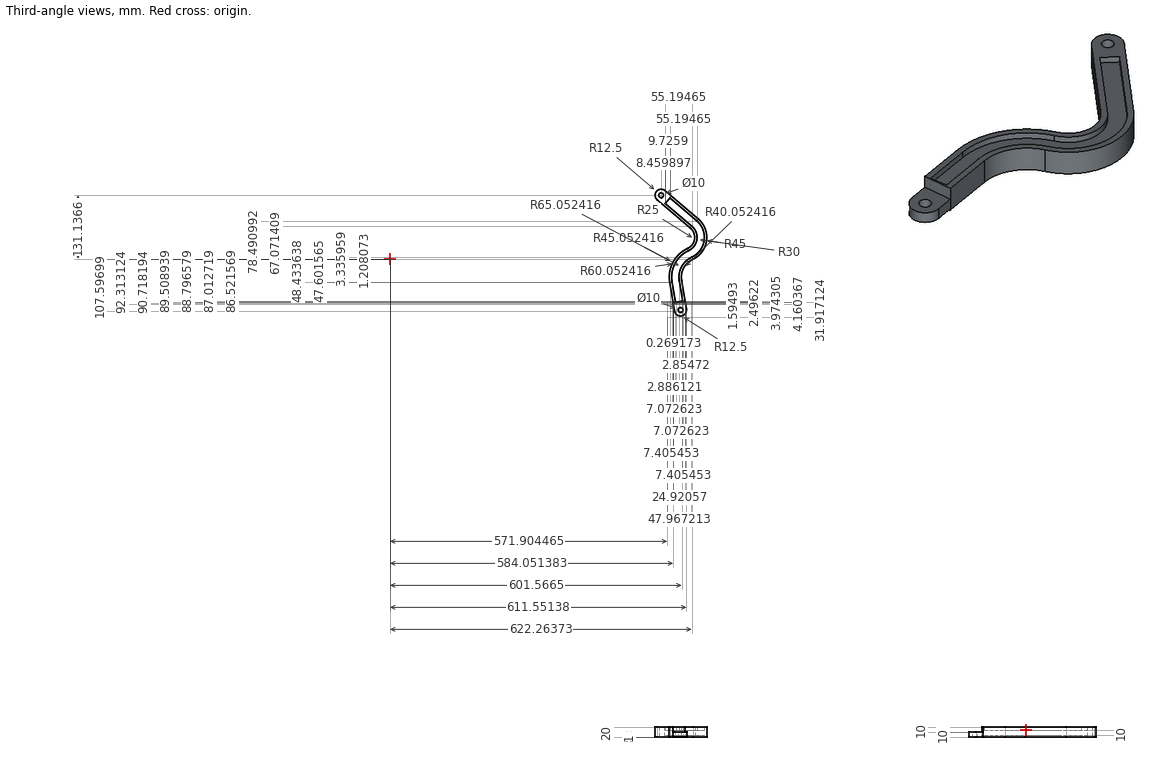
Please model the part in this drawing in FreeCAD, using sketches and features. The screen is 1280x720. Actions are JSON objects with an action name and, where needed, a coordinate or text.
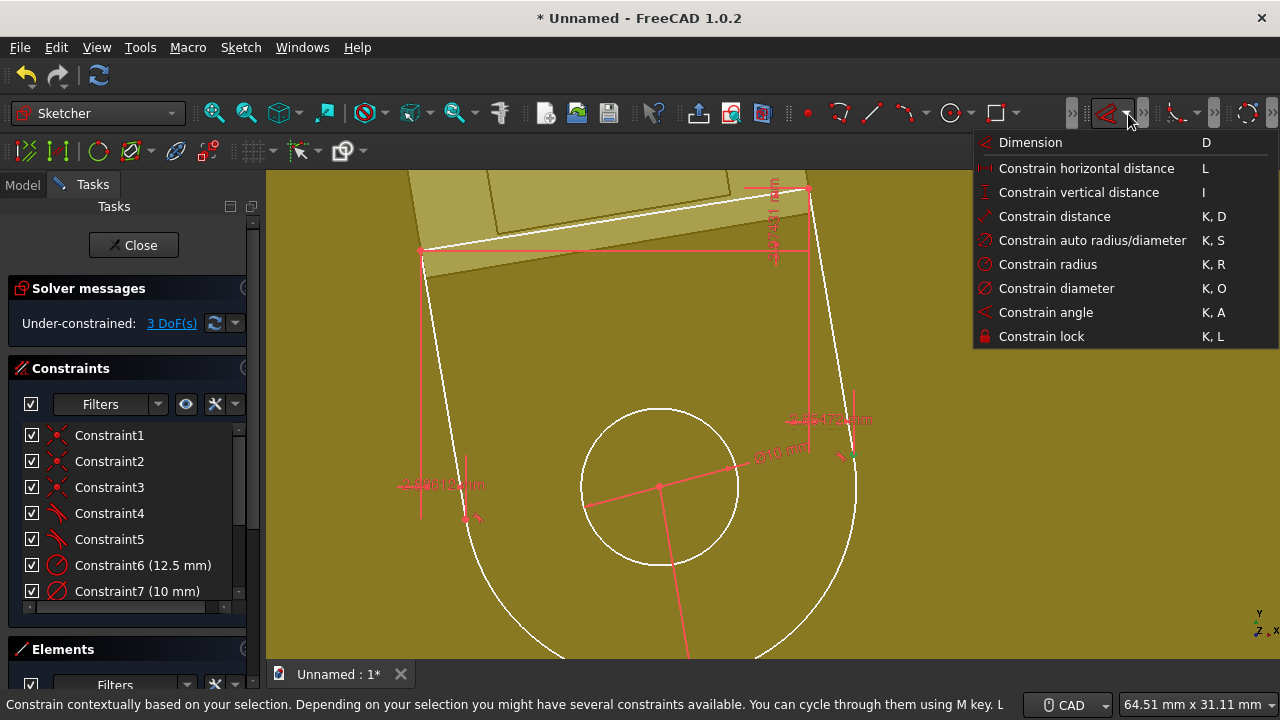
{"action": "left_click", "coordinate": [1126, 168]}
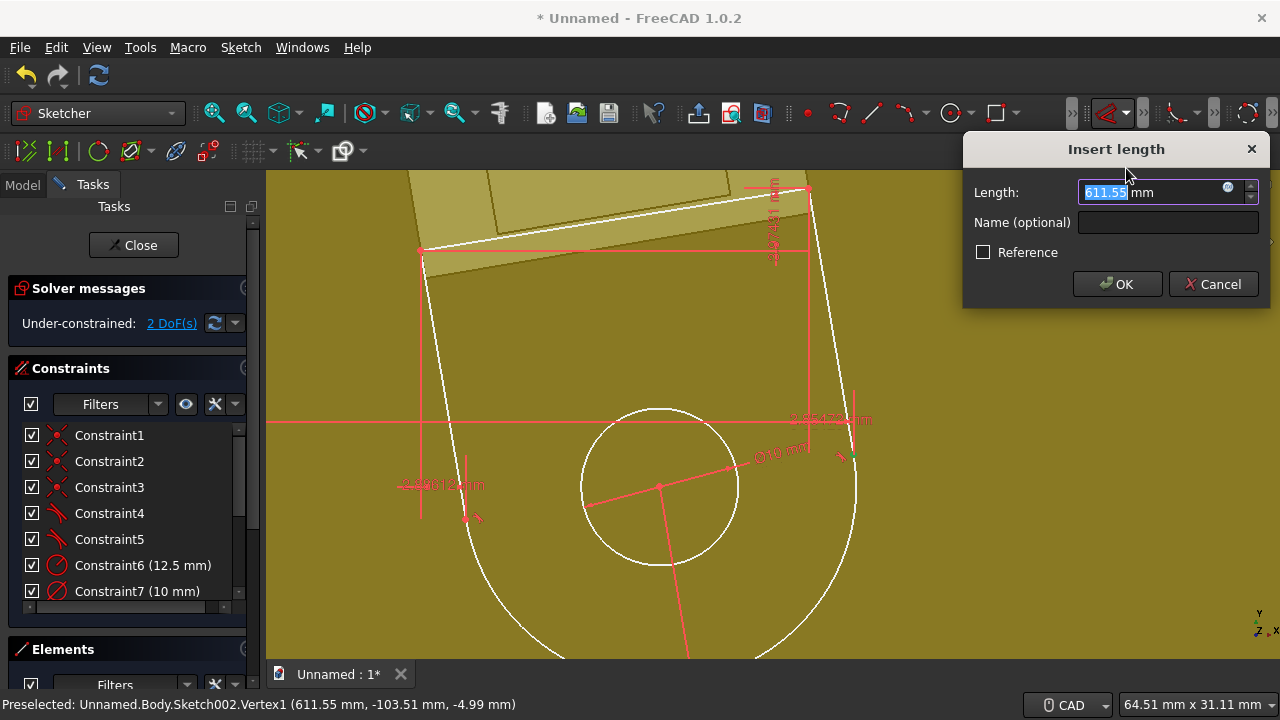
{"action": "type", "text": "611.55138"}
{"action": "key", "text": "Return"}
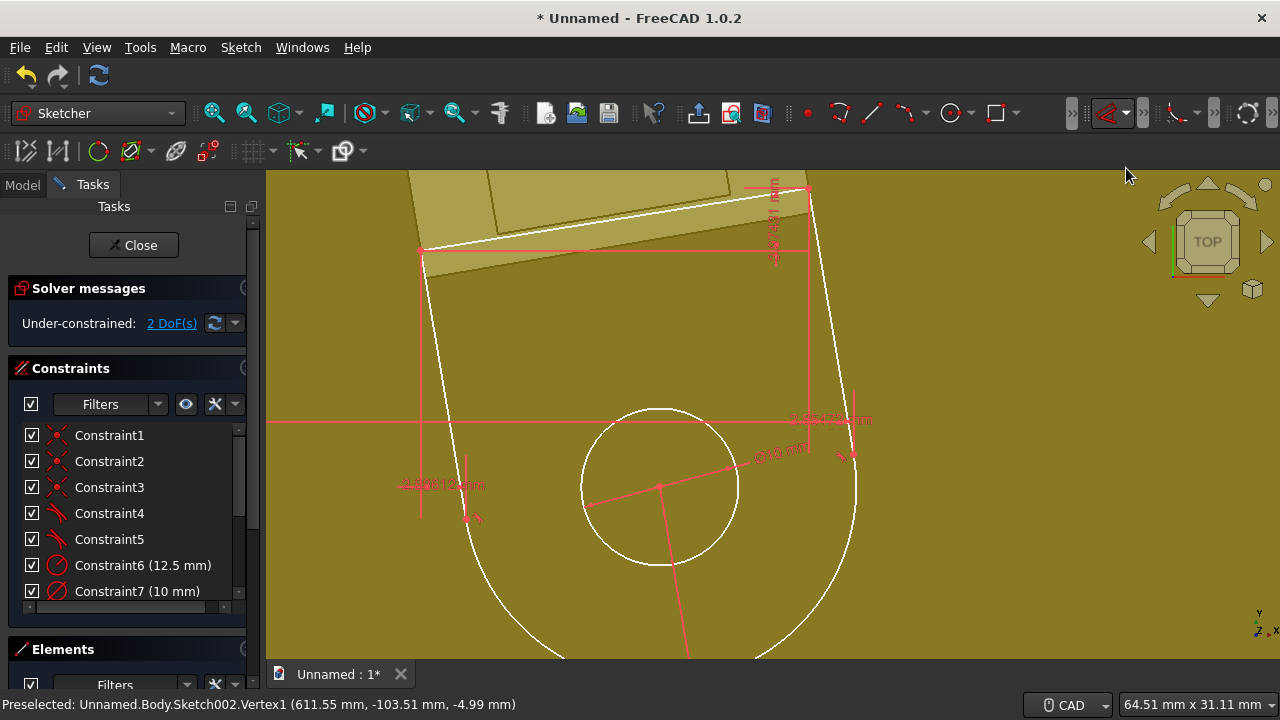
{"action": "scroll", "coordinate": [841, 376], "scroll_direction": "down", "scroll_amount": 2}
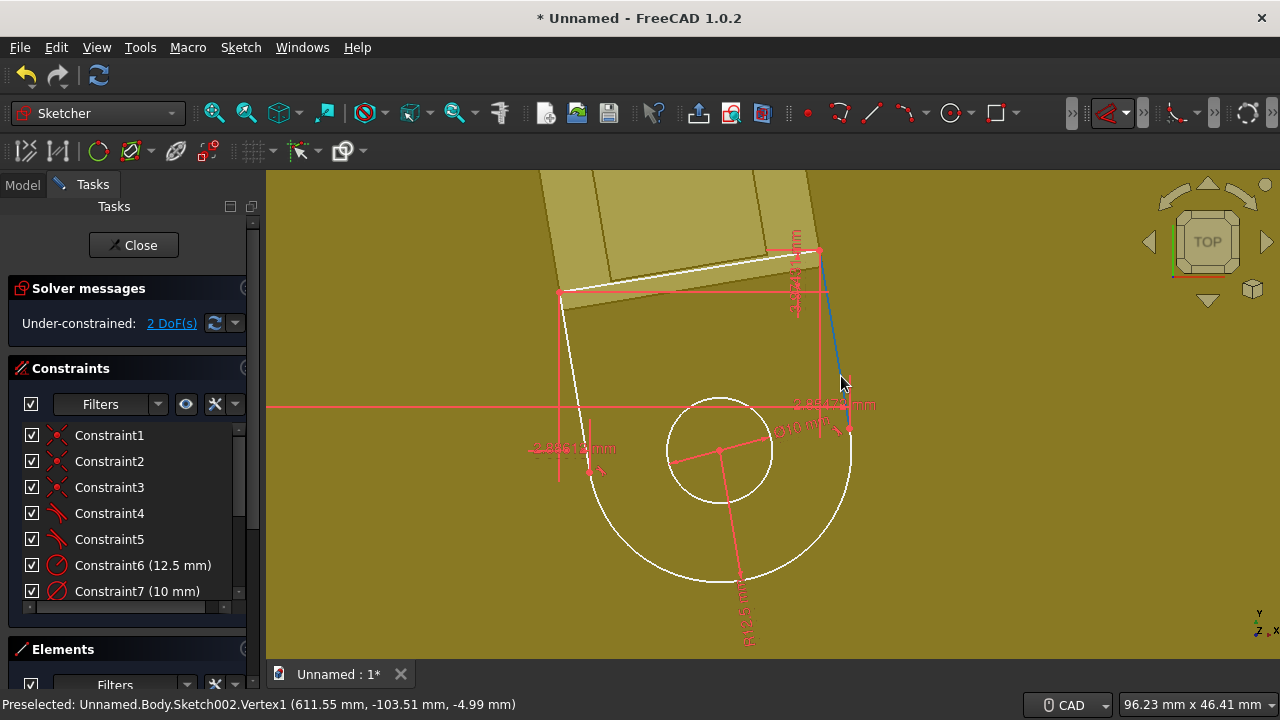
{"action": "left_click", "coordinate": [820, 250]}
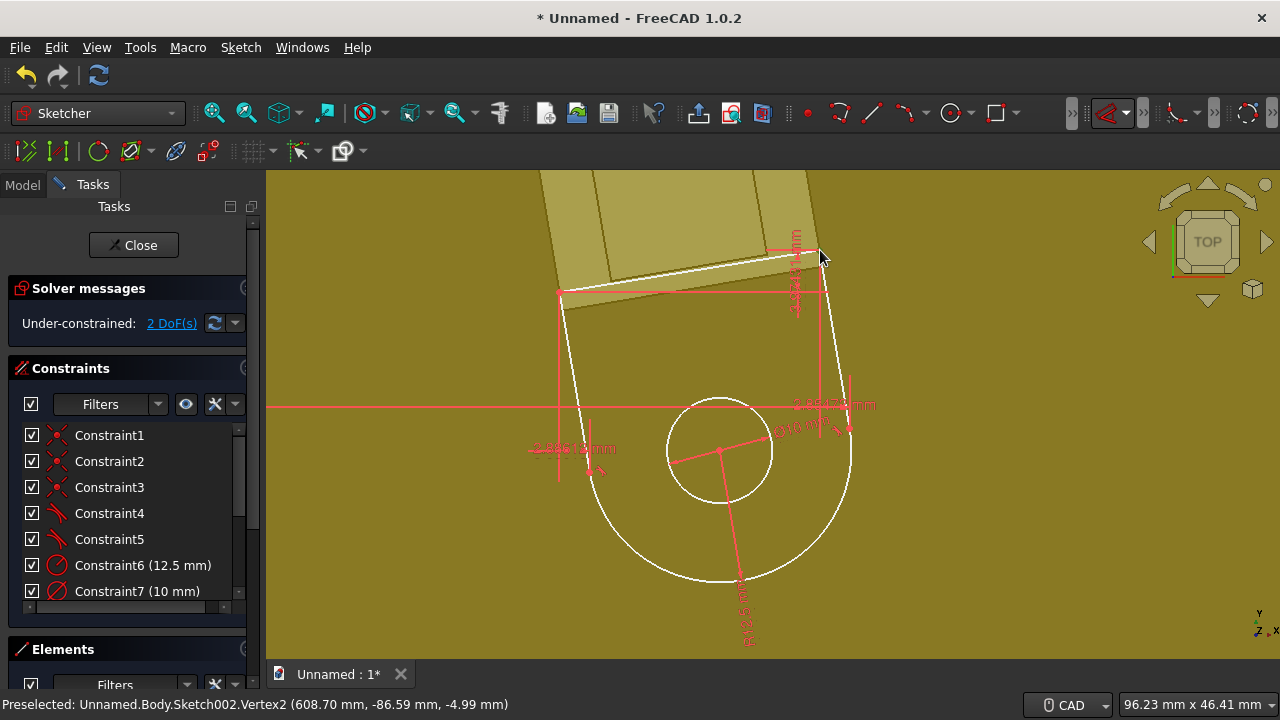
{"action": "key", "text": "i"}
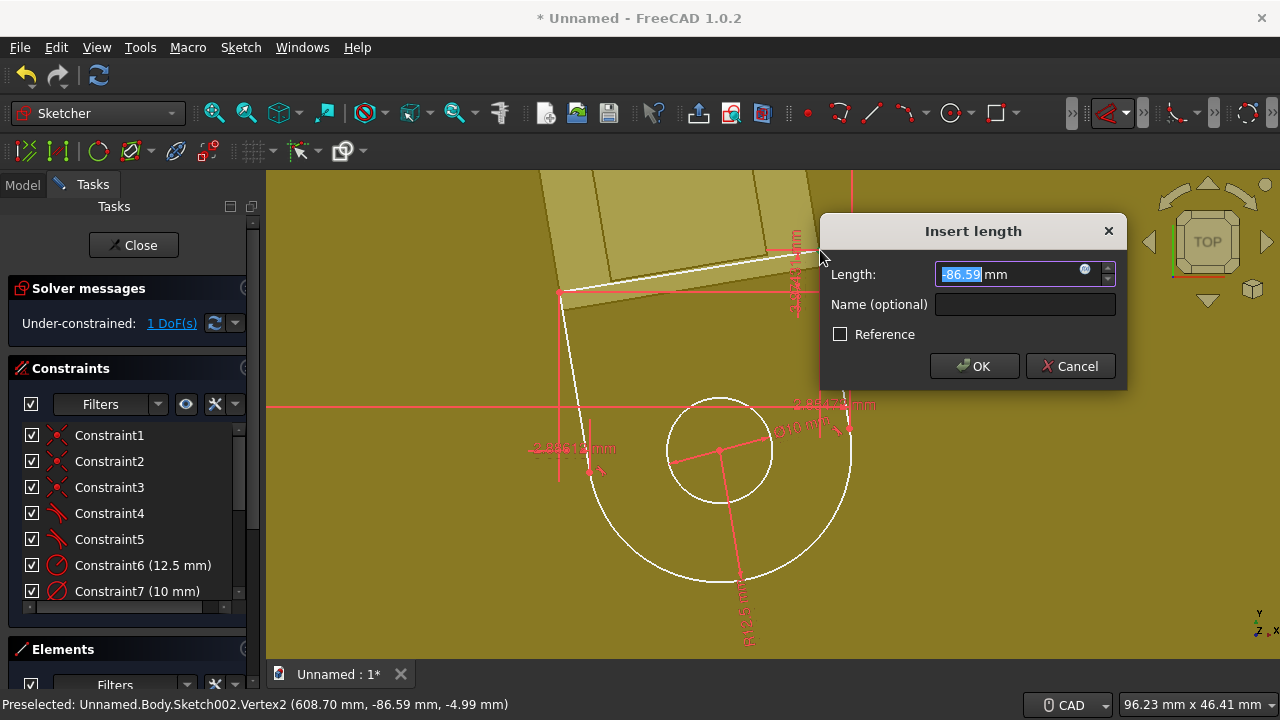
{"action": "type", "text": "-86.521569"}
{"action": "key", "text": "Return"}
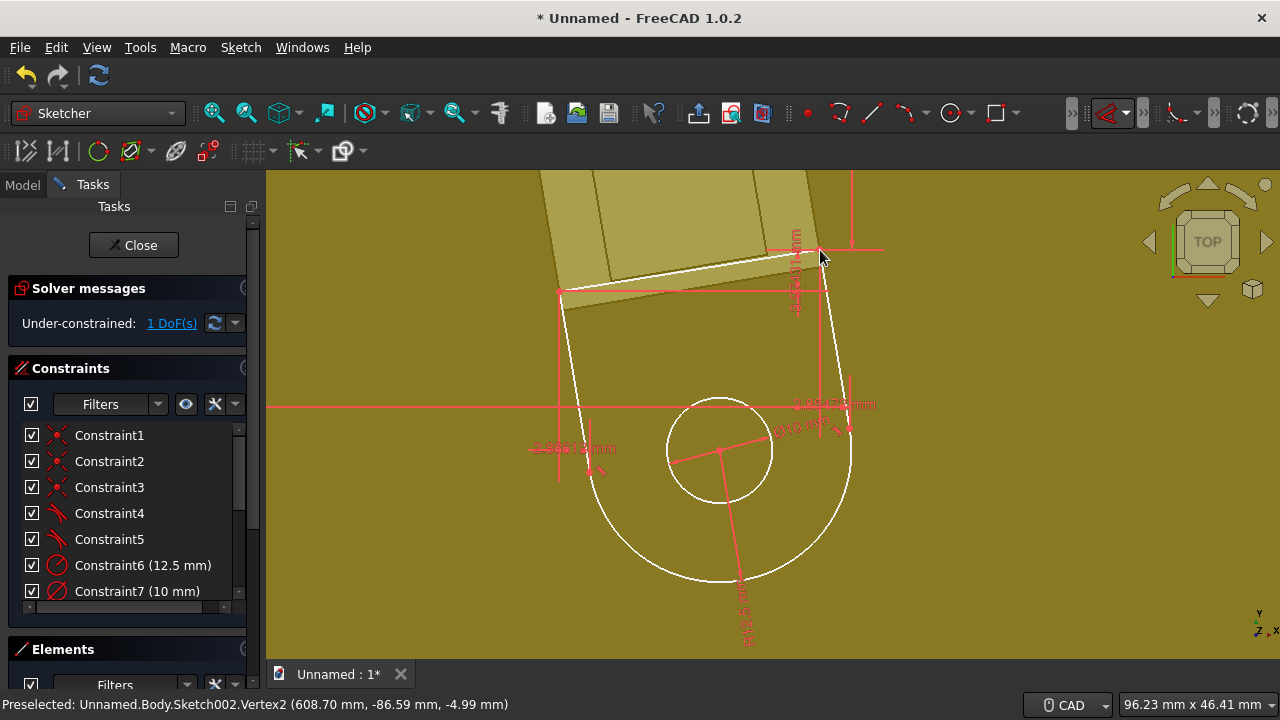
{"action": "left_click", "coordinate": [590, 472]}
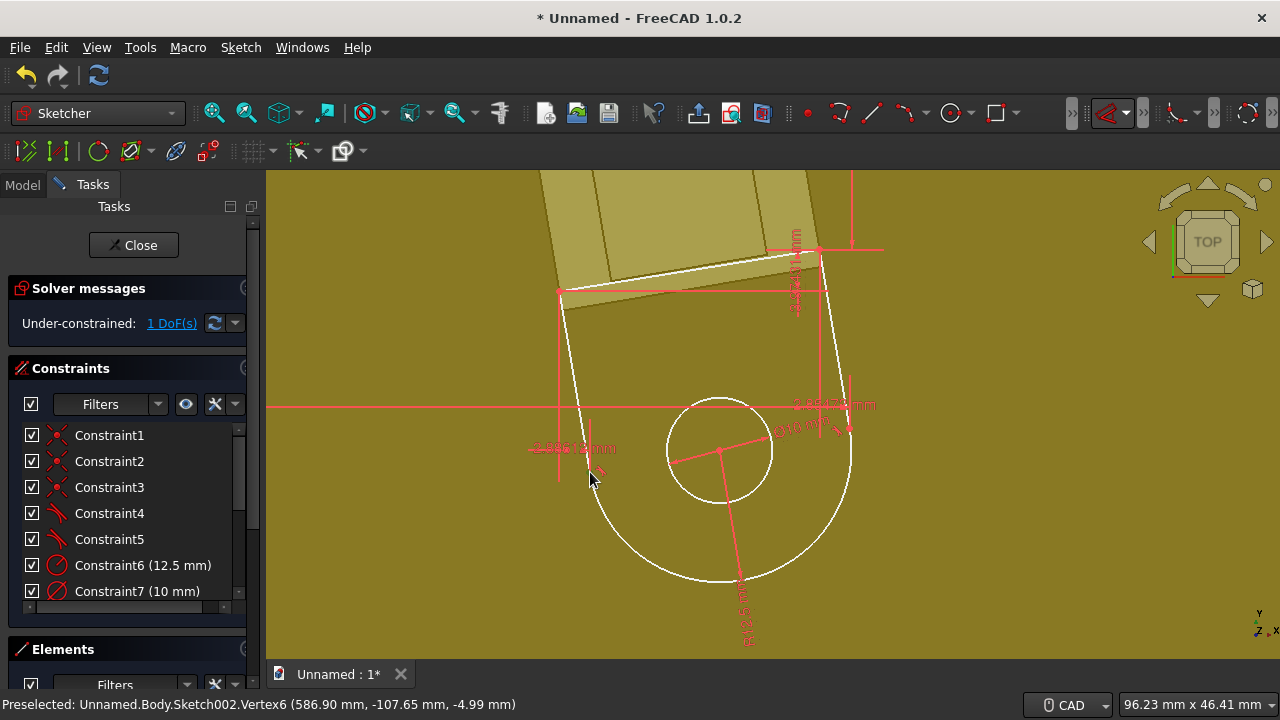
{"action": "key", "text": "i"}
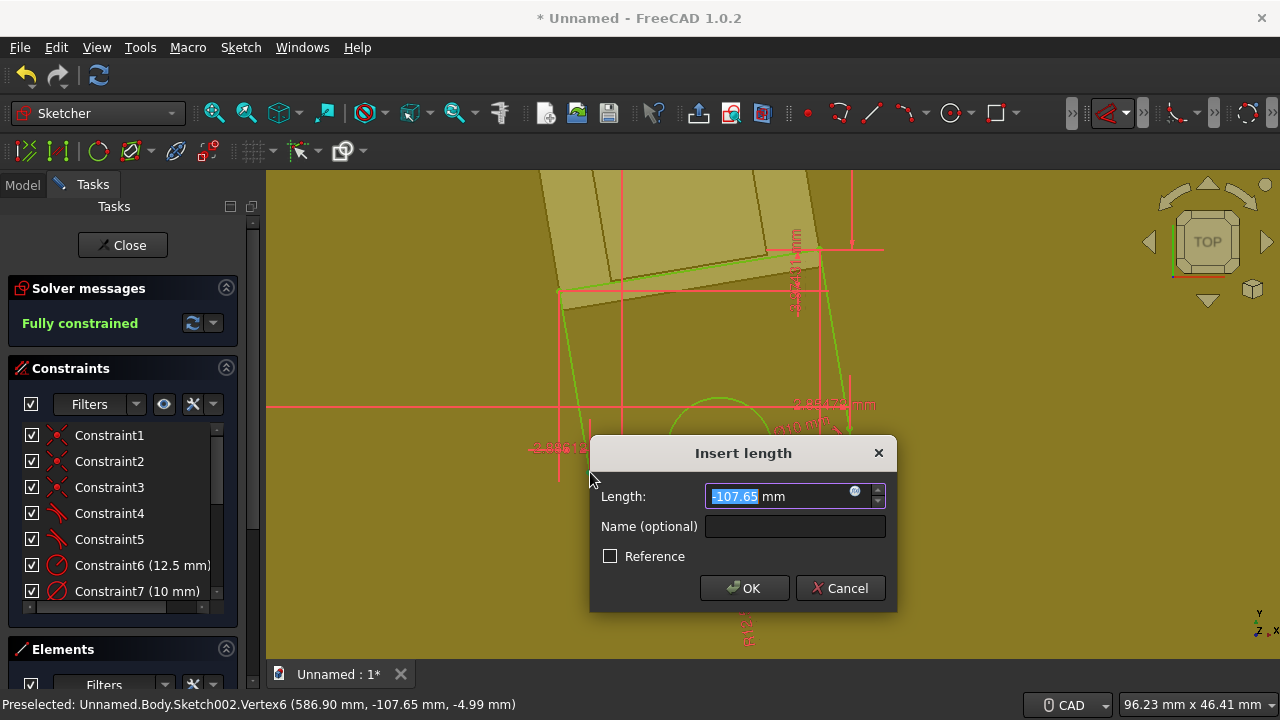
{"action": "type", "text": "-107.59699"}
{"action": "key", "text": "Return"}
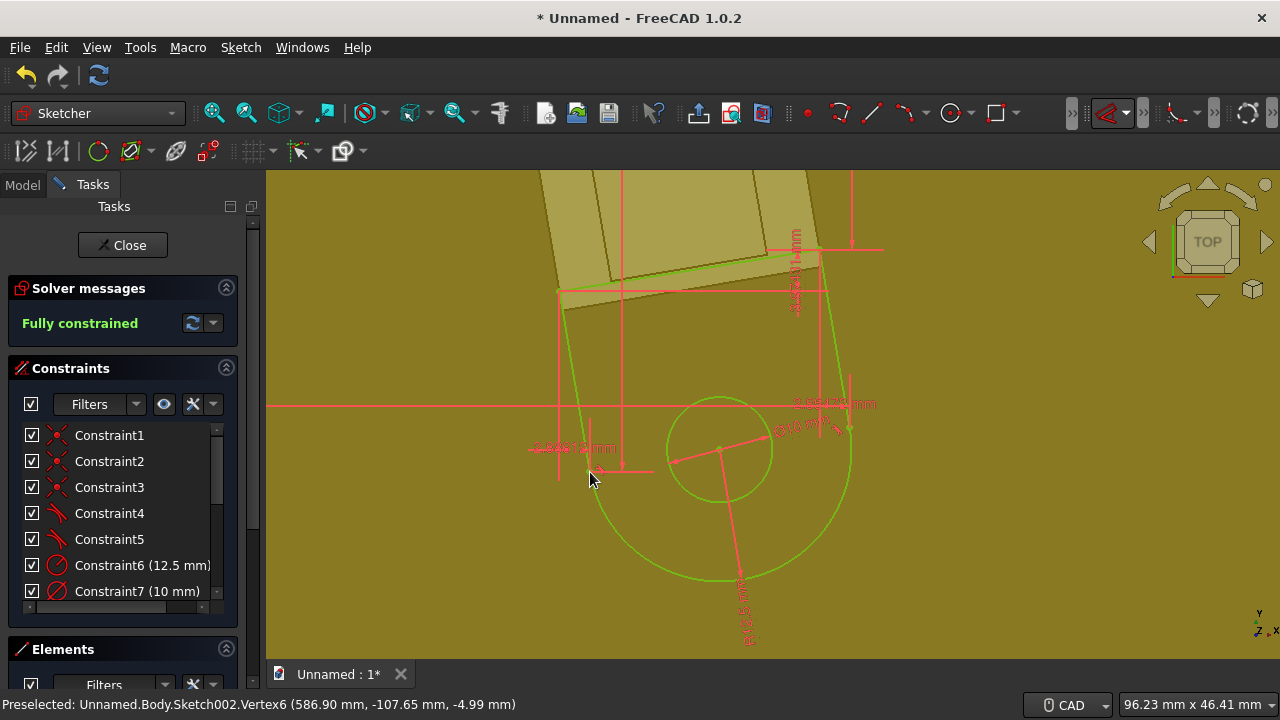
{"action": "left_click", "coordinate": [123, 245]}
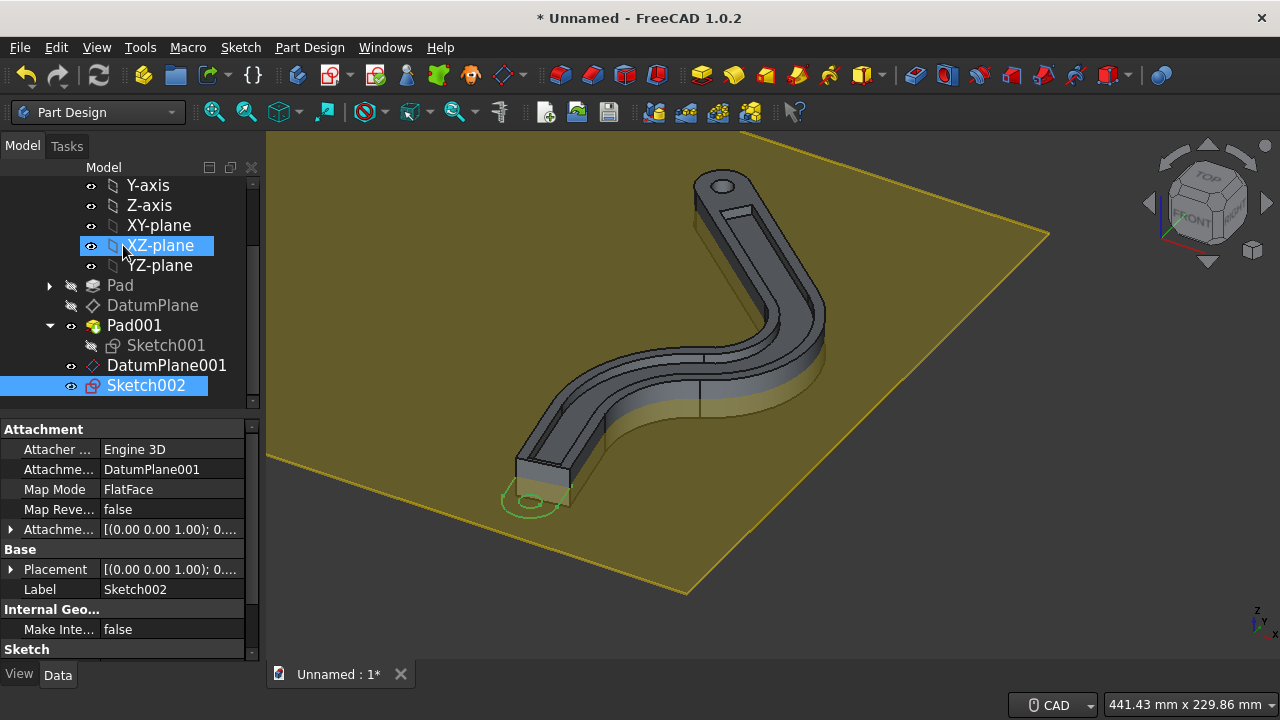
{"action": "left_click", "coordinate": [702, 76]}